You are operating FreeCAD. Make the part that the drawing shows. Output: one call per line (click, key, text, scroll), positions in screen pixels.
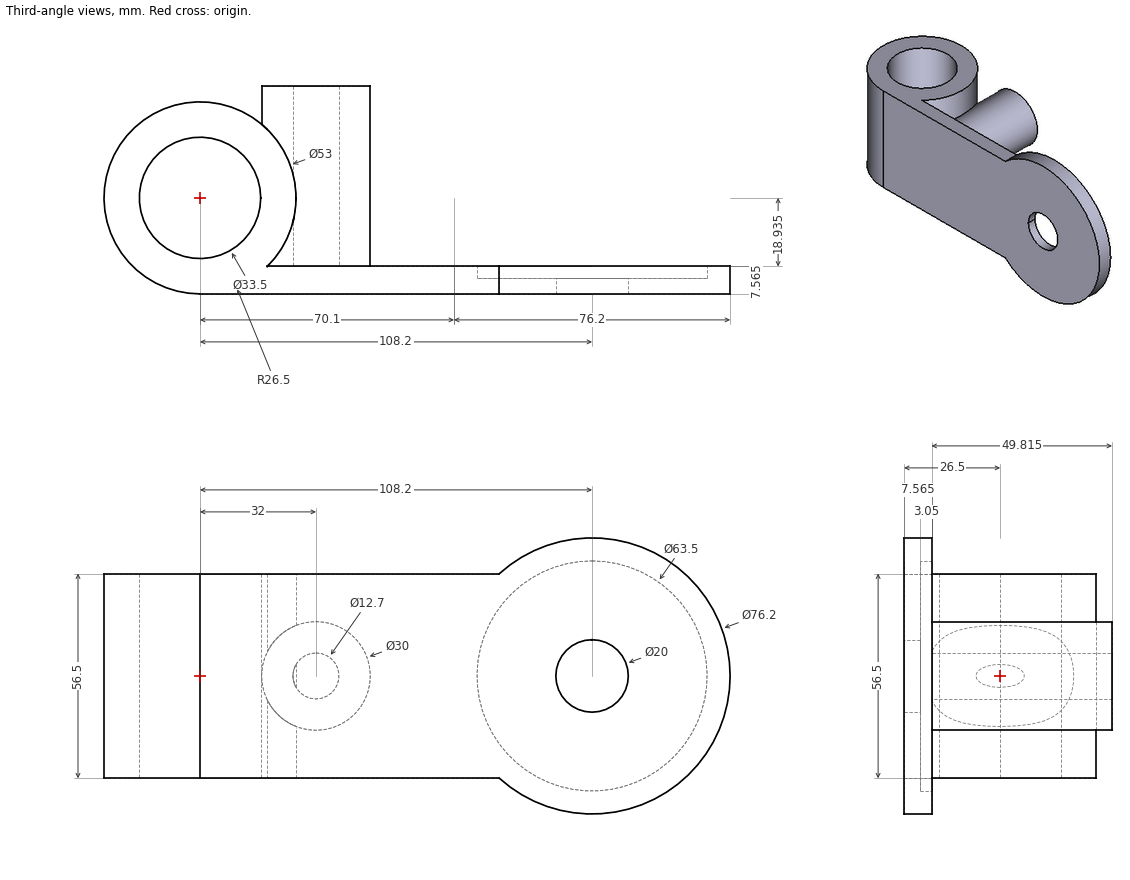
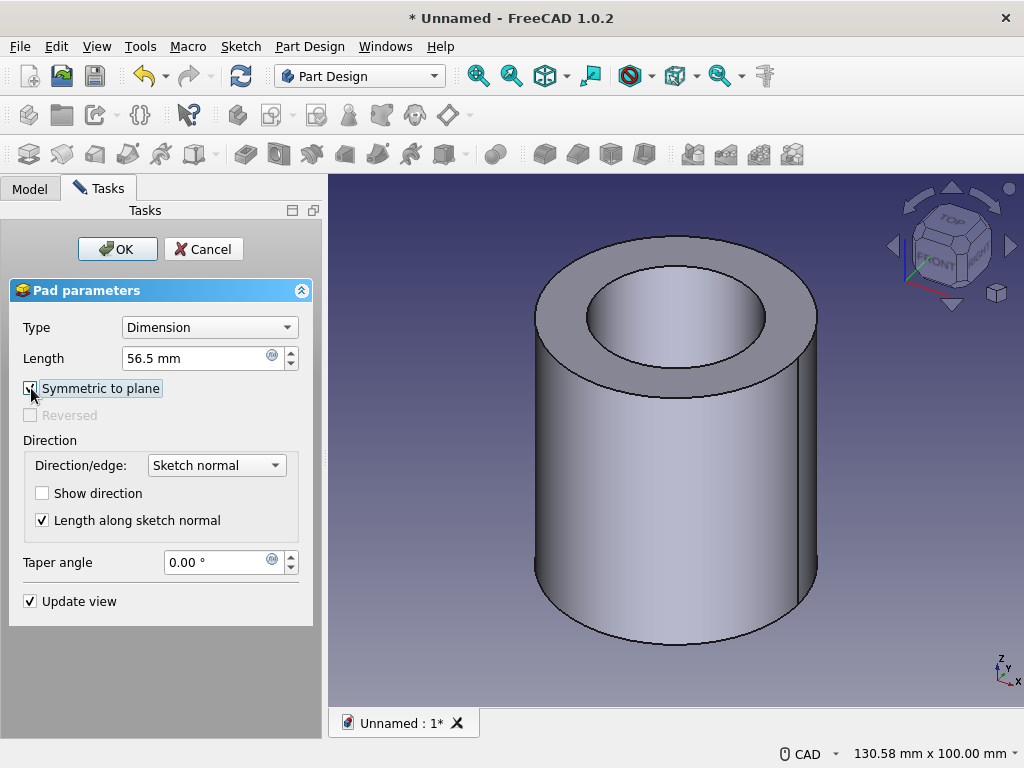
click(118, 249)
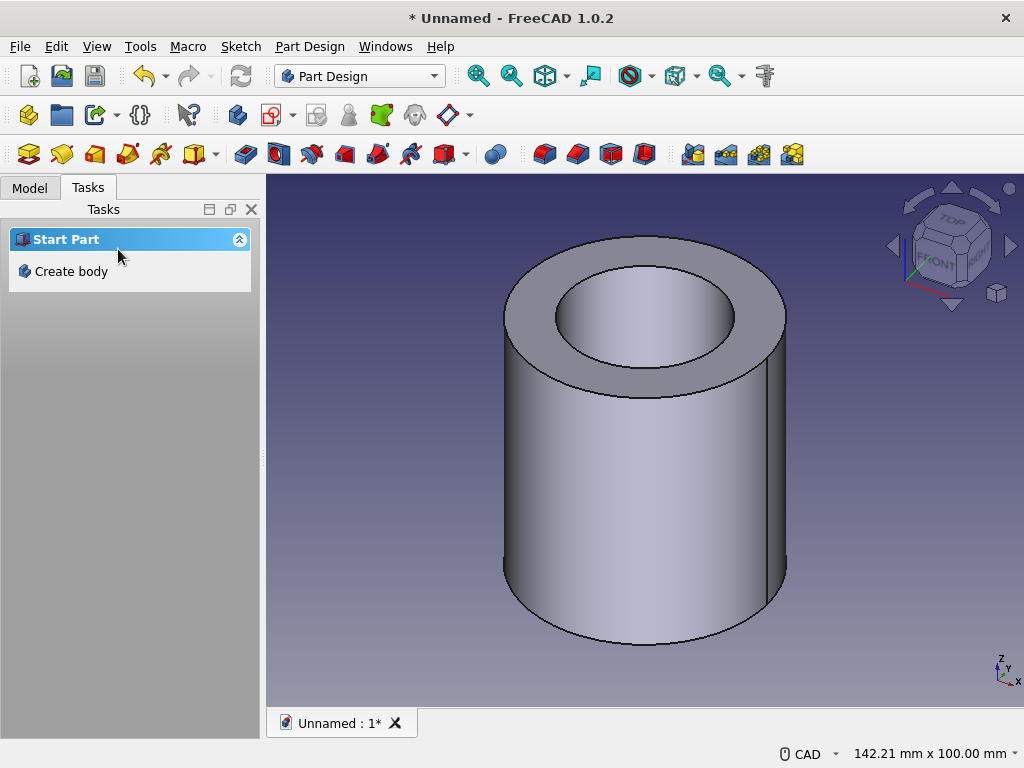
click(270, 116)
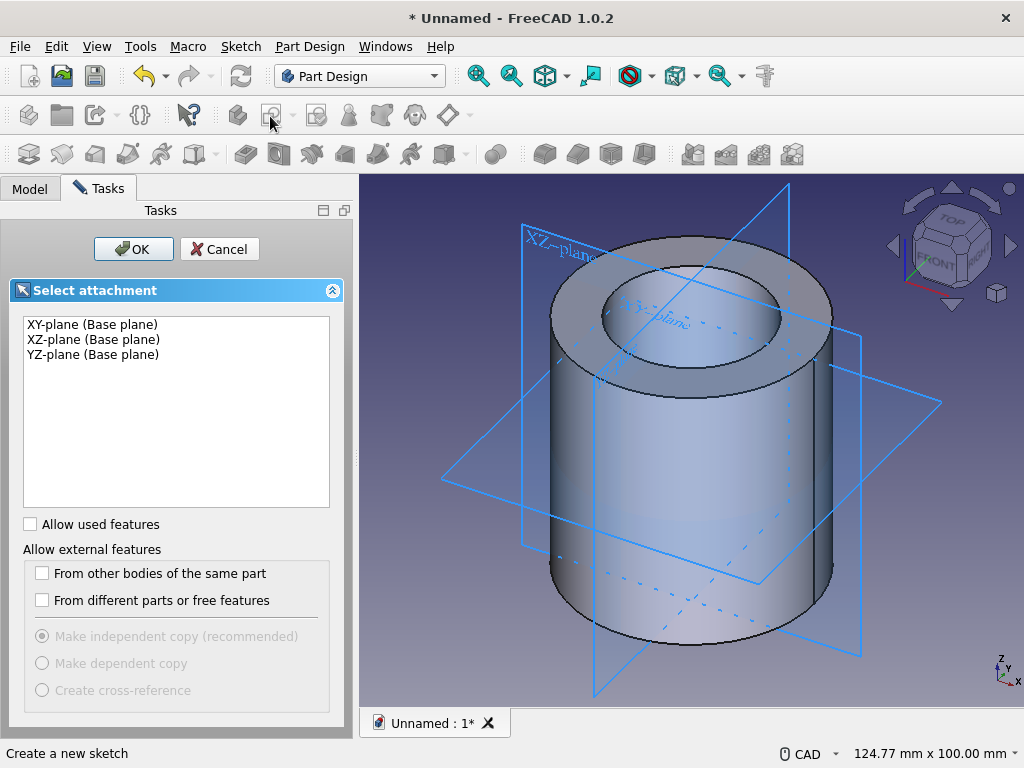
click(84, 324)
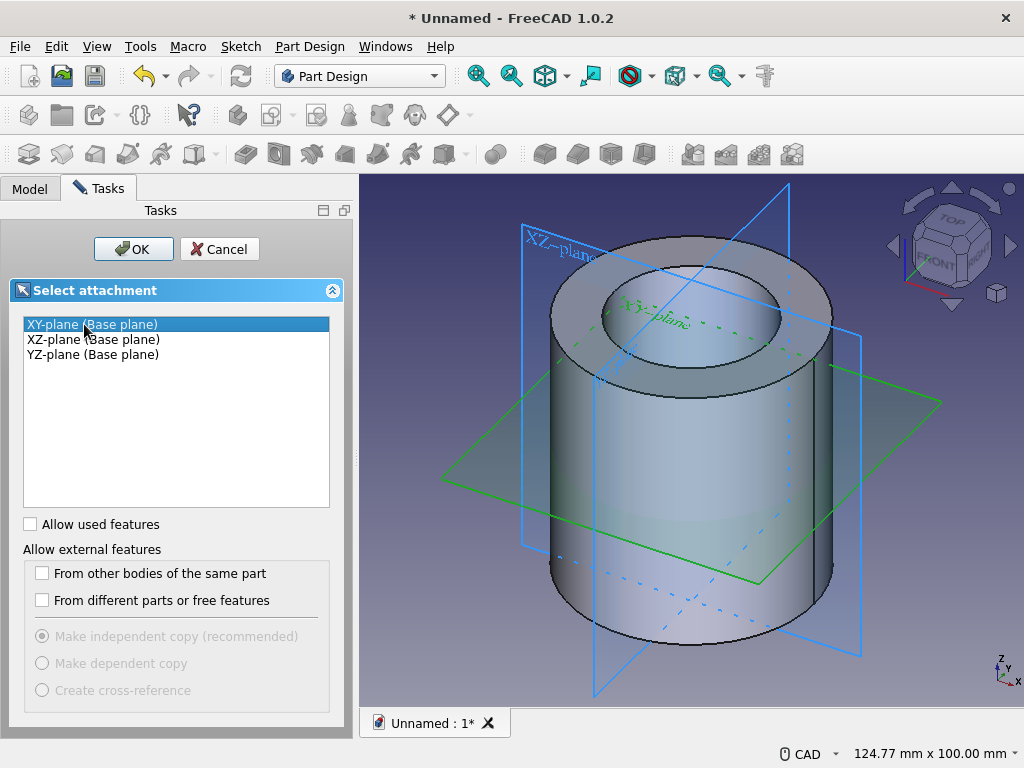
click(134, 249)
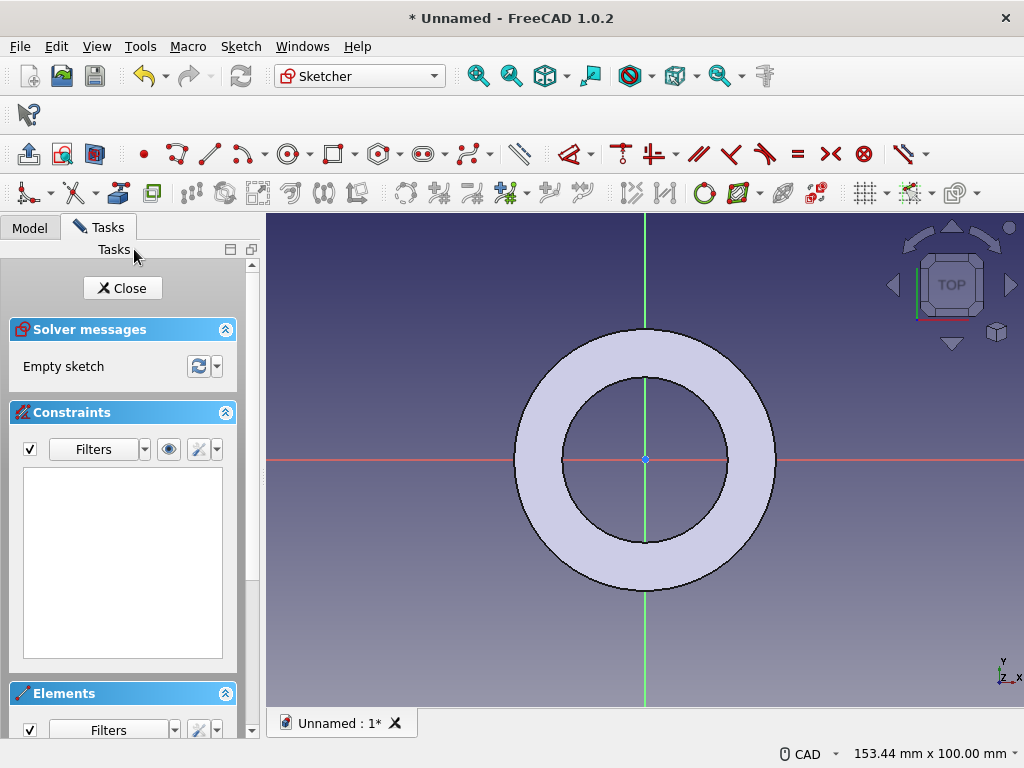
key(q)
key(s)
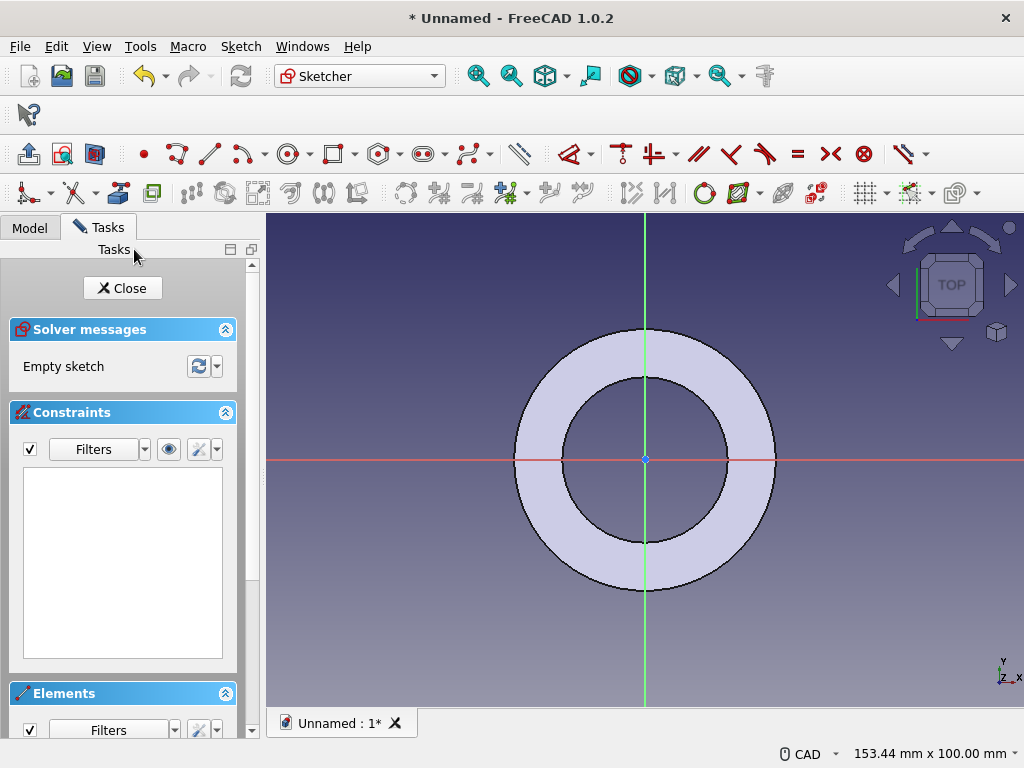
scroll(294, 380, down, 3)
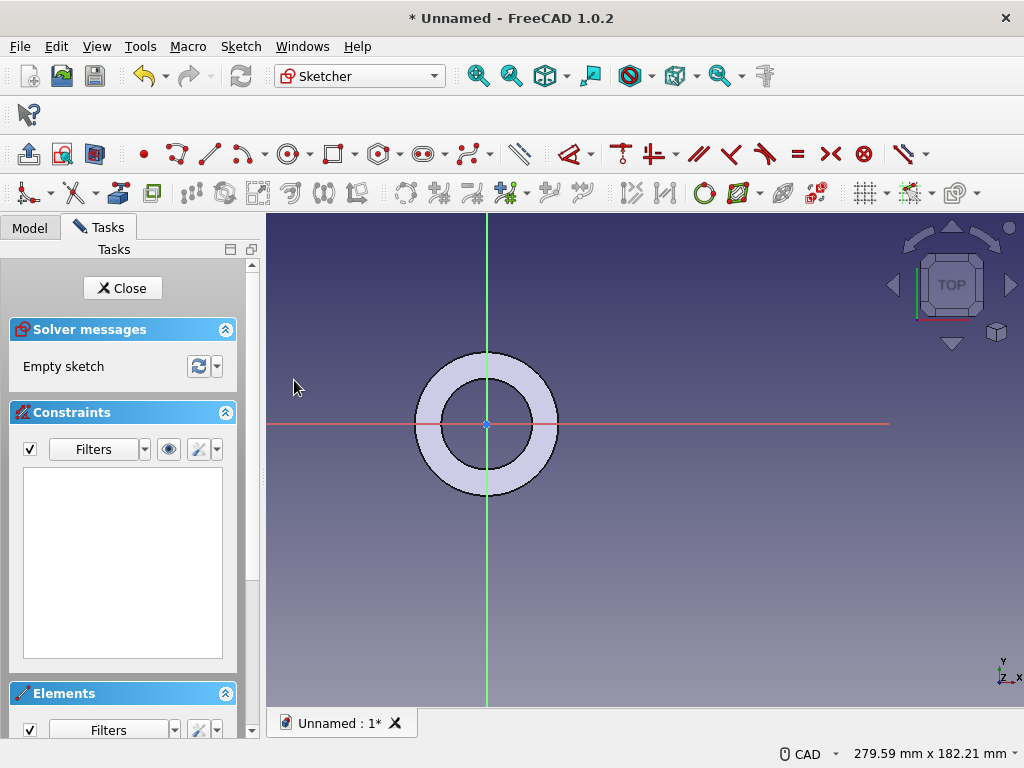
scroll(749, 460, up, 2)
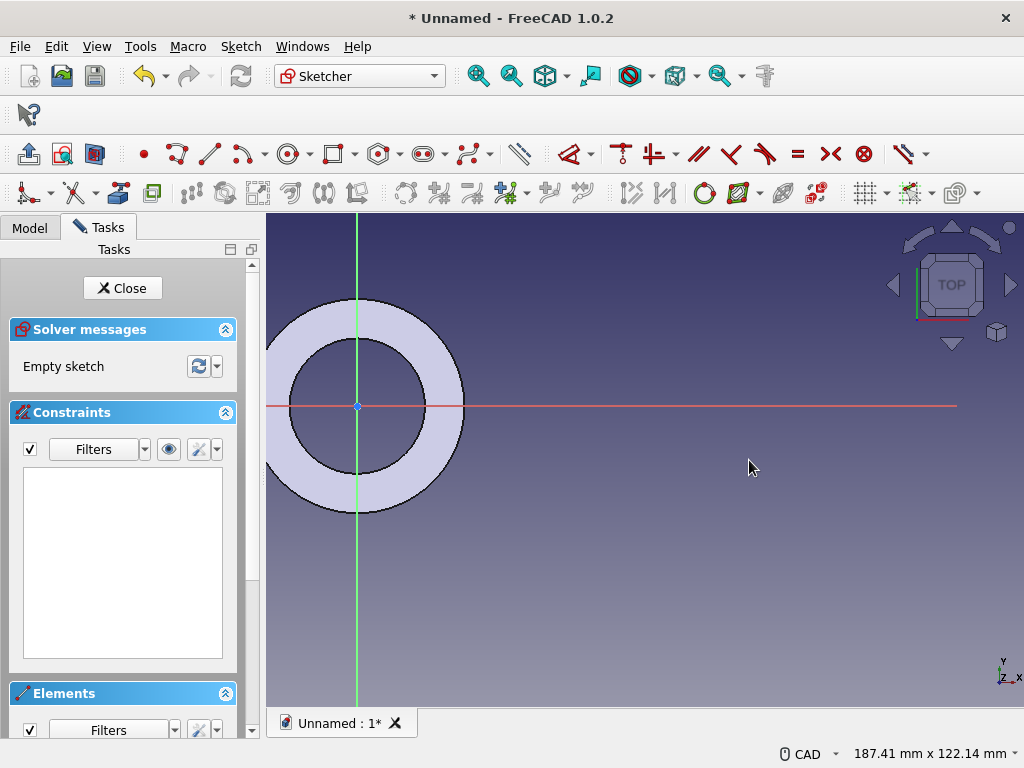
click(177, 154)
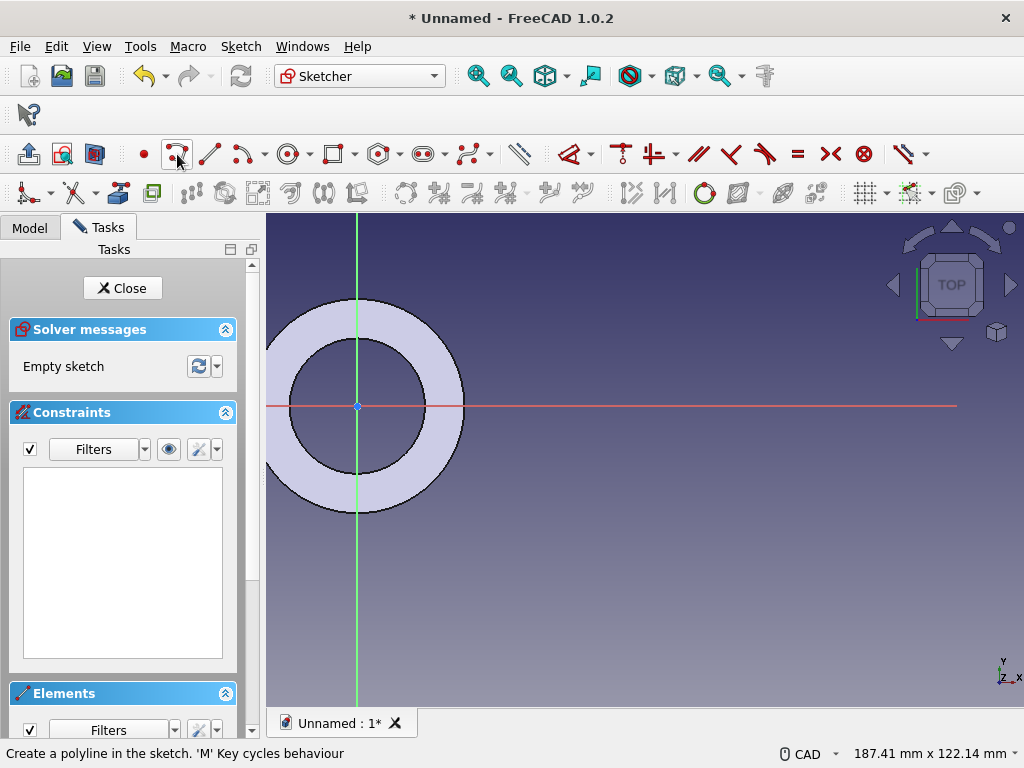
click(357, 513)
click(795, 513)
click(795, 483)
click(432, 483)
right_click(432, 483)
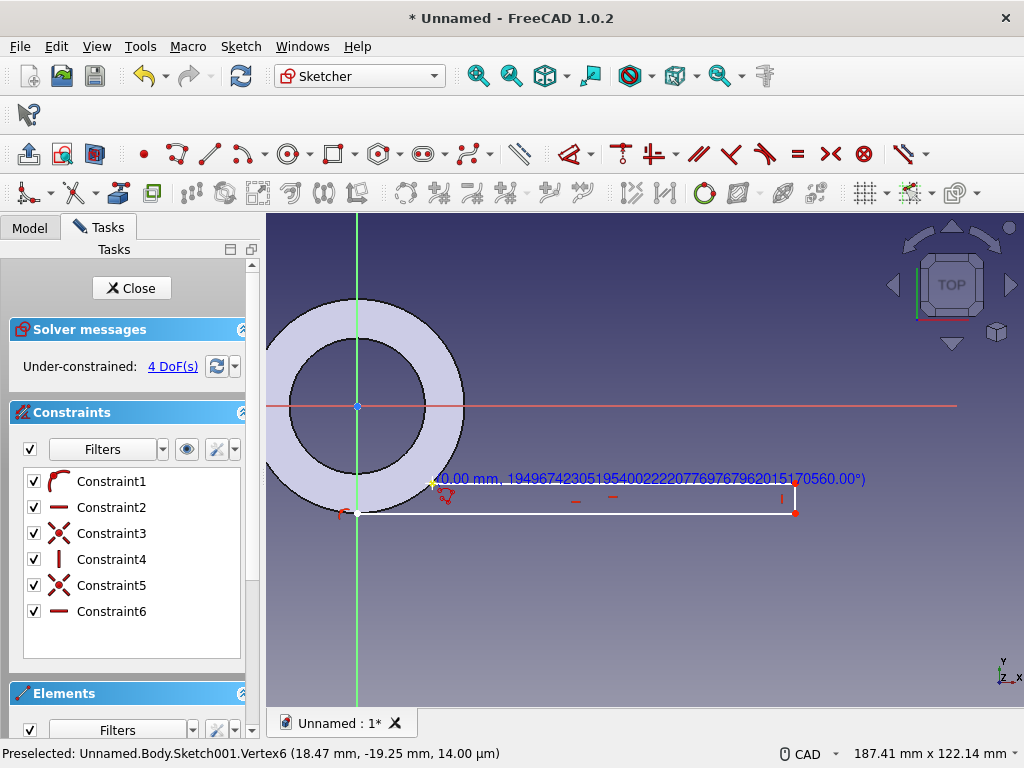
key(g)
key(3)
key(a)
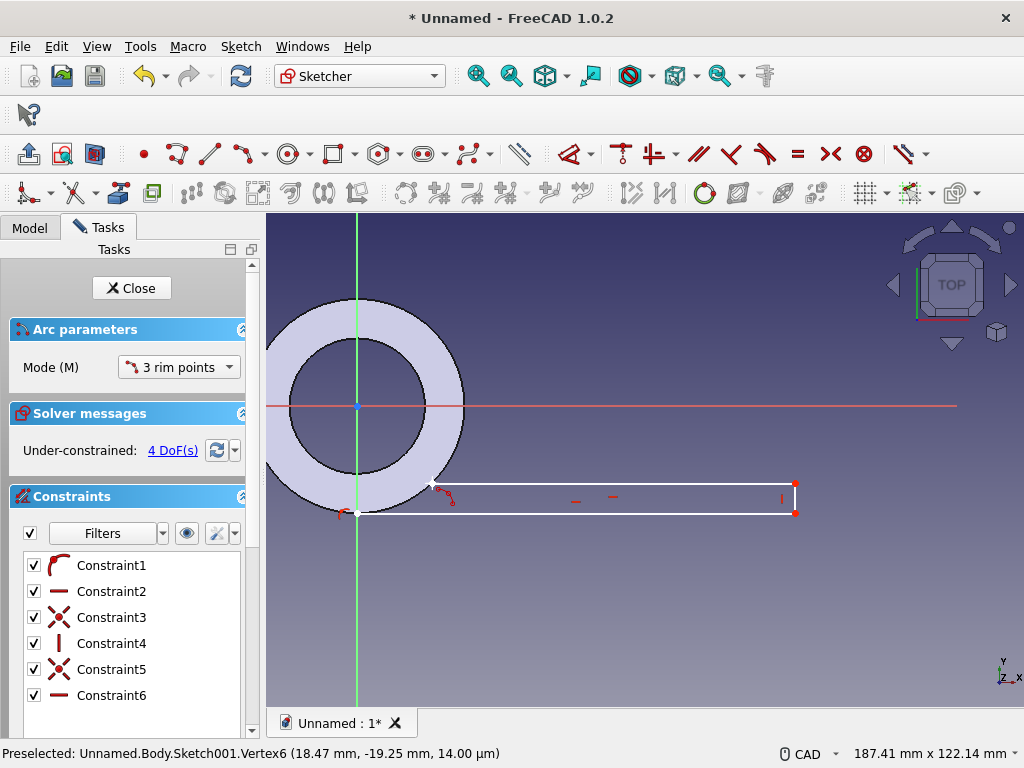
click(432, 484)
click(357, 514)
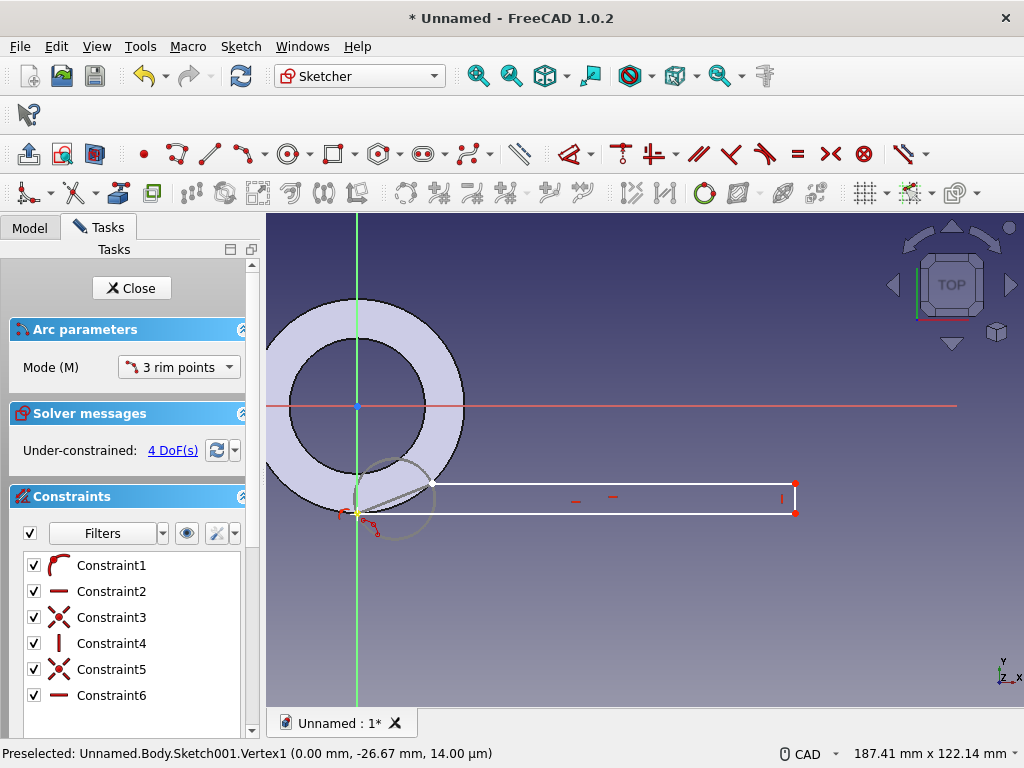
scroll(398, 505, up, 4)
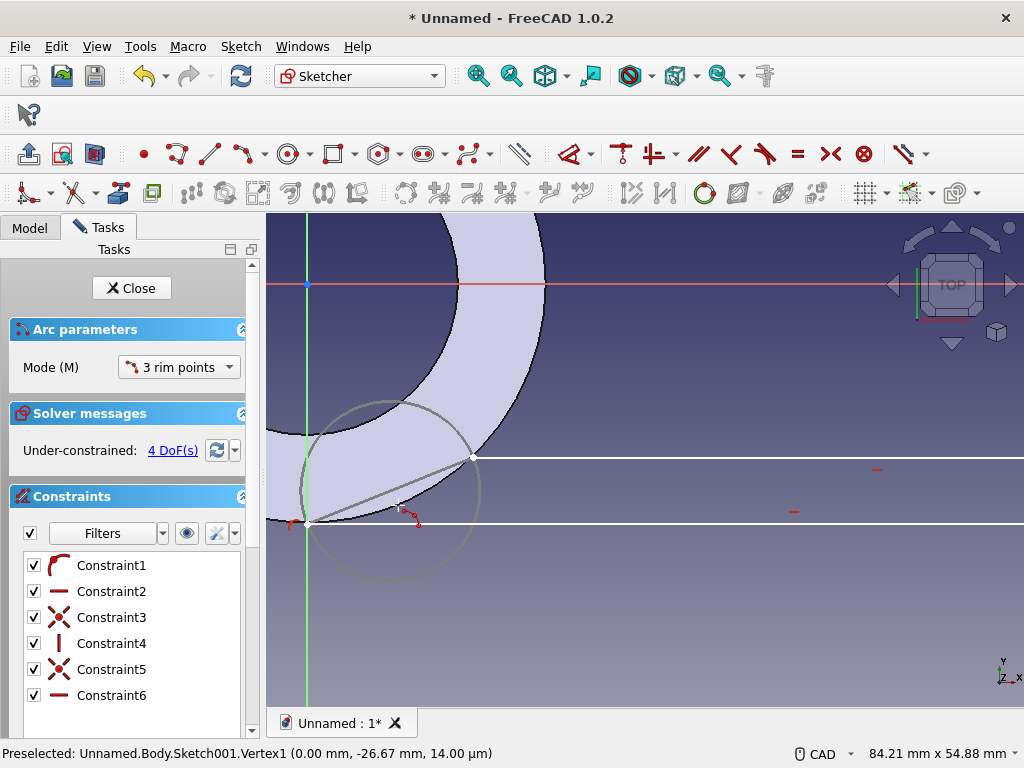
click(397, 505)
key(Escape)